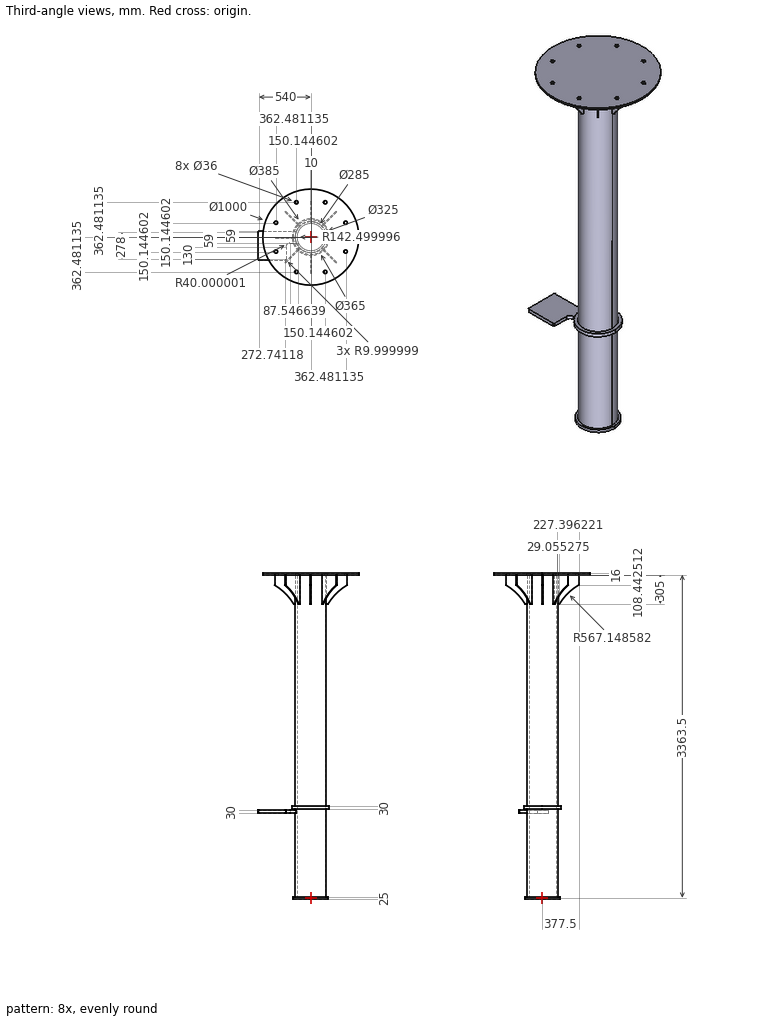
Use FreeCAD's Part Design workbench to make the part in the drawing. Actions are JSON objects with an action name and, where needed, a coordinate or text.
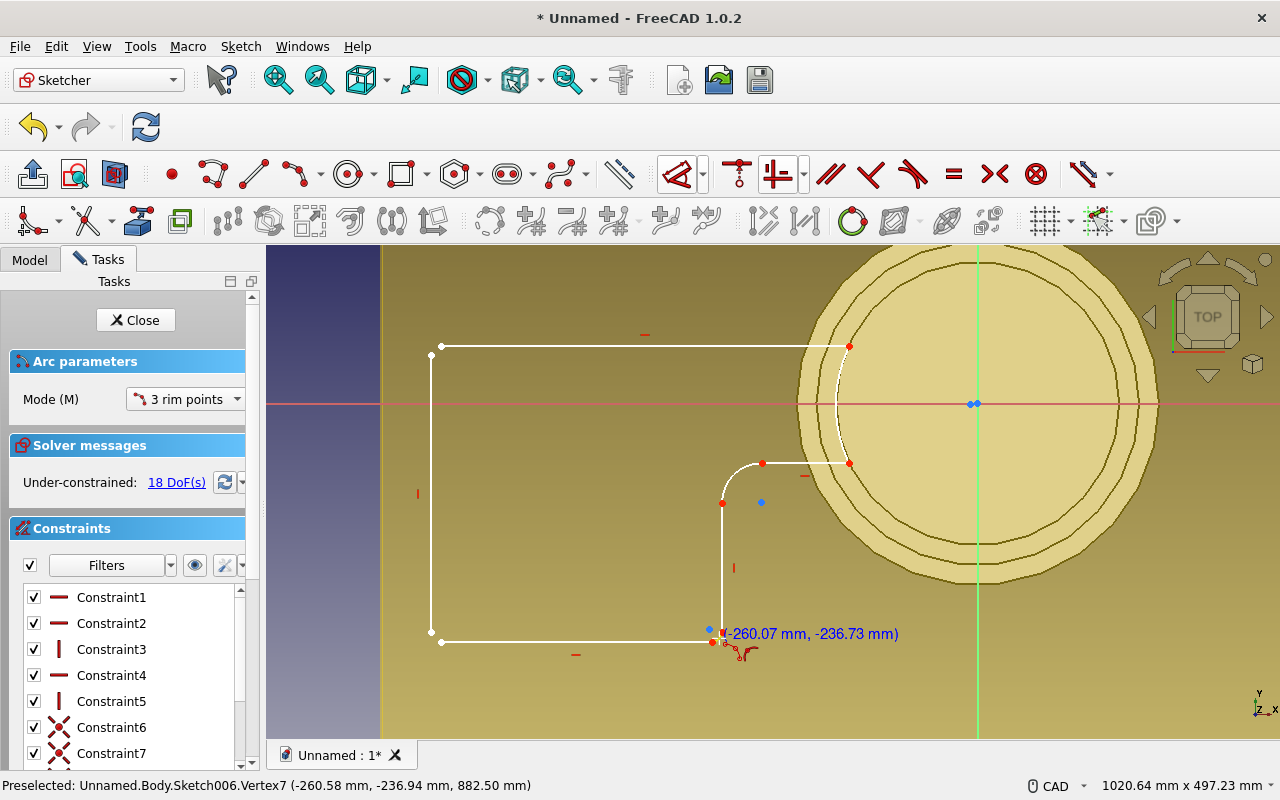
{"action": "left_click", "coordinate": [441, 642]}
{"action": "left_click", "coordinate": [431, 632]}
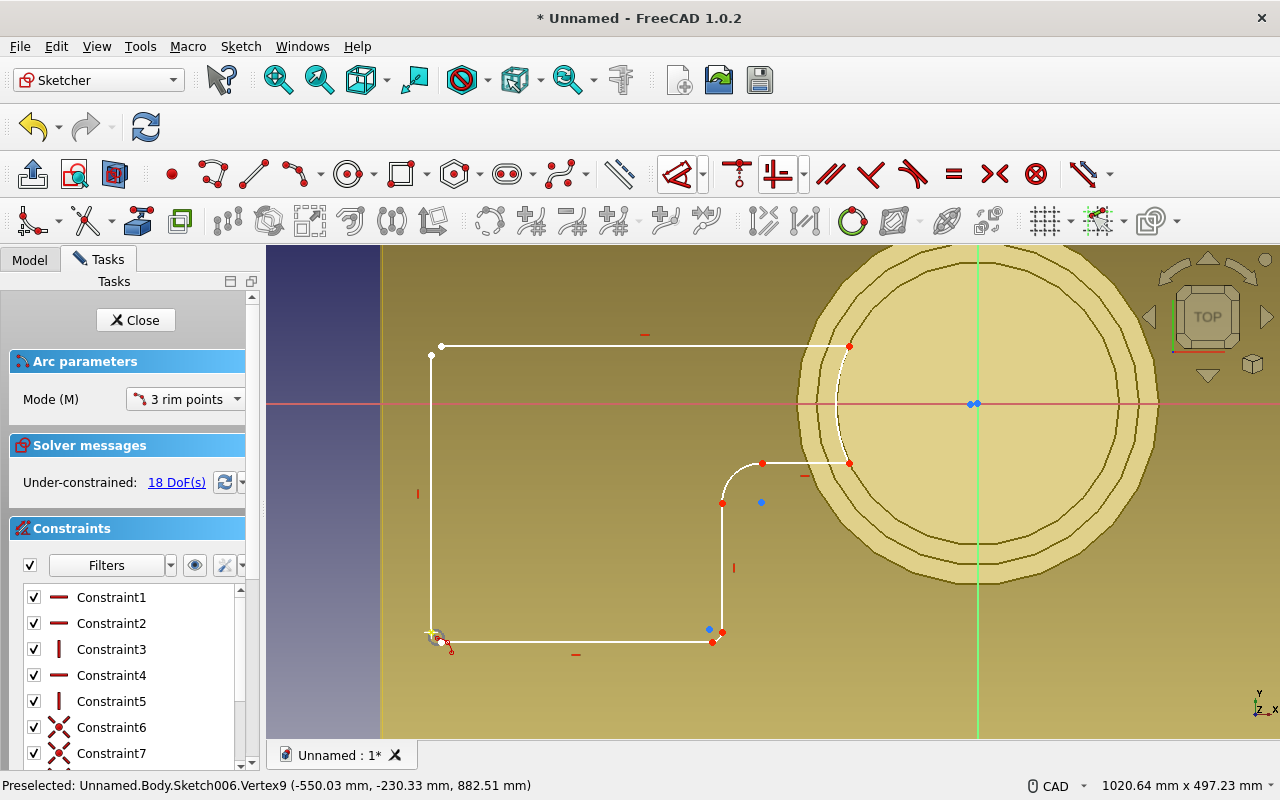
{"action": "scroll", "coordinate": [434, 638], "scroll_direction": "up", "scroll_amount": 9}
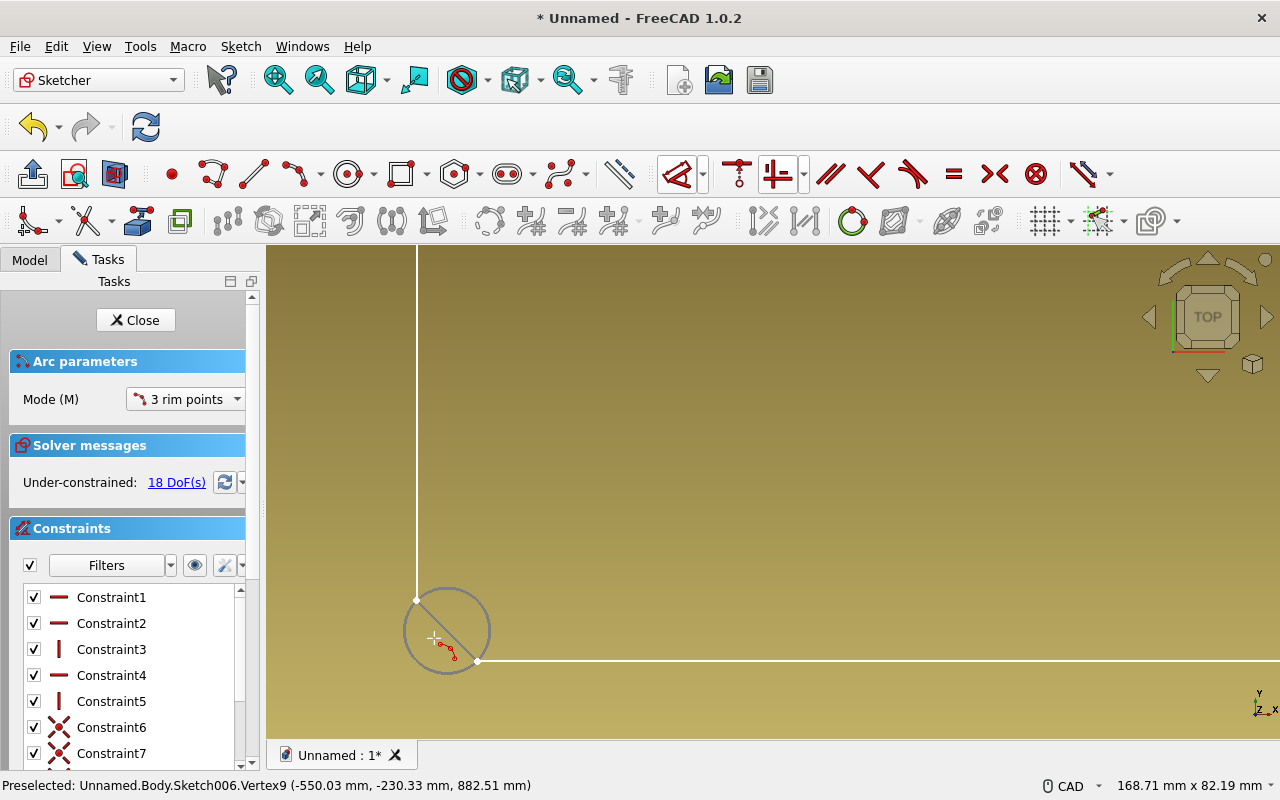
{"action": "left_click", "coordinate": [435, 635]}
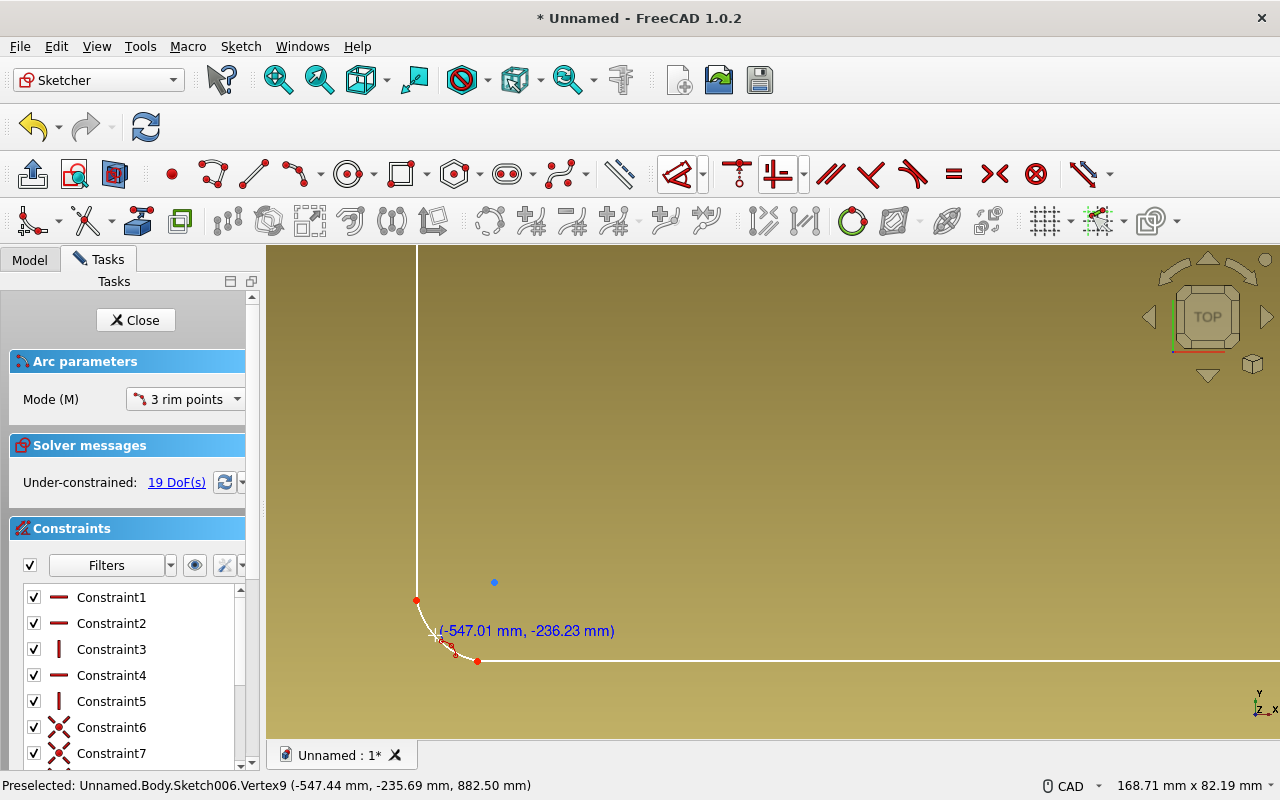
{"action": "scroll", "coordinate": [434, 638], "scroll_direction": "down", "scroll_amount": 9}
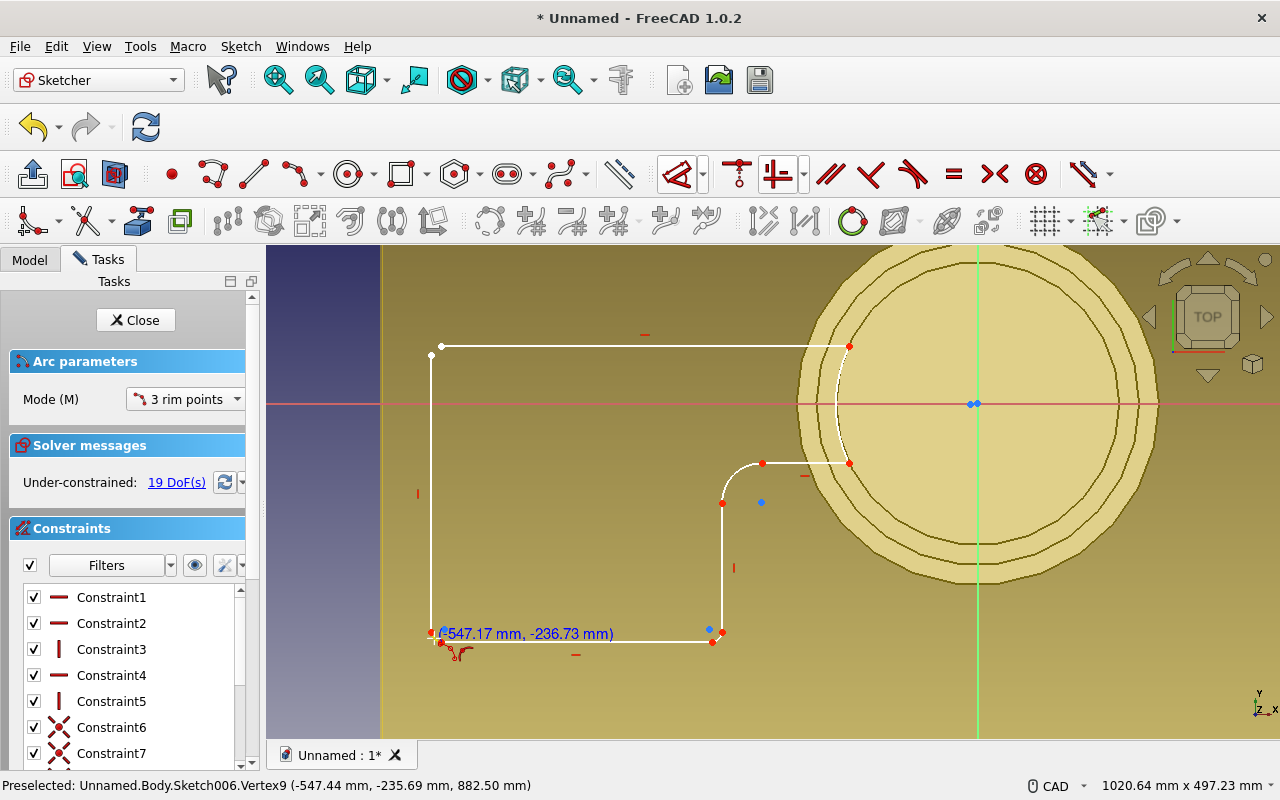
{"action": "left_click", "coordinate": [431, 355]}
{"action": "left_click", "coordinate": [441, 346]}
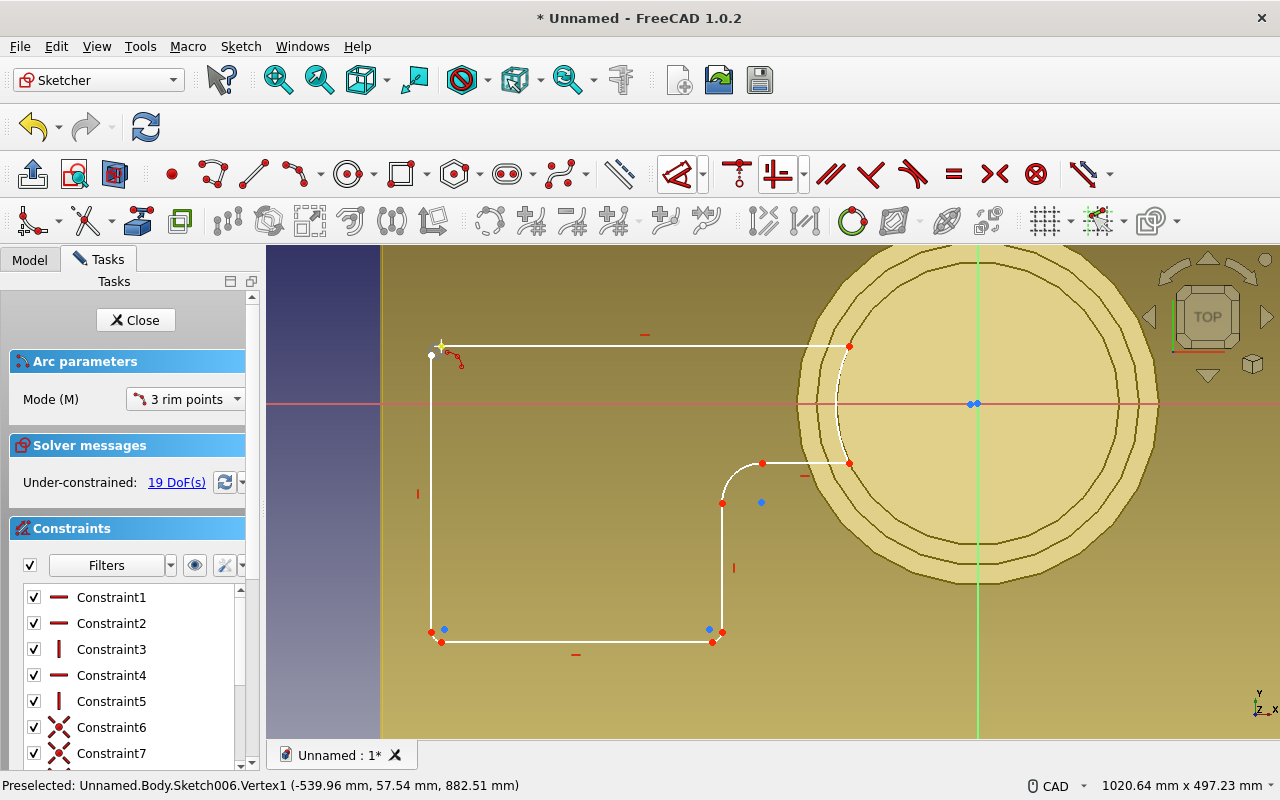
{"action": "scroll", "coordinate": [434, 348], "scroll_direction": "up", "scroll_amount": 9}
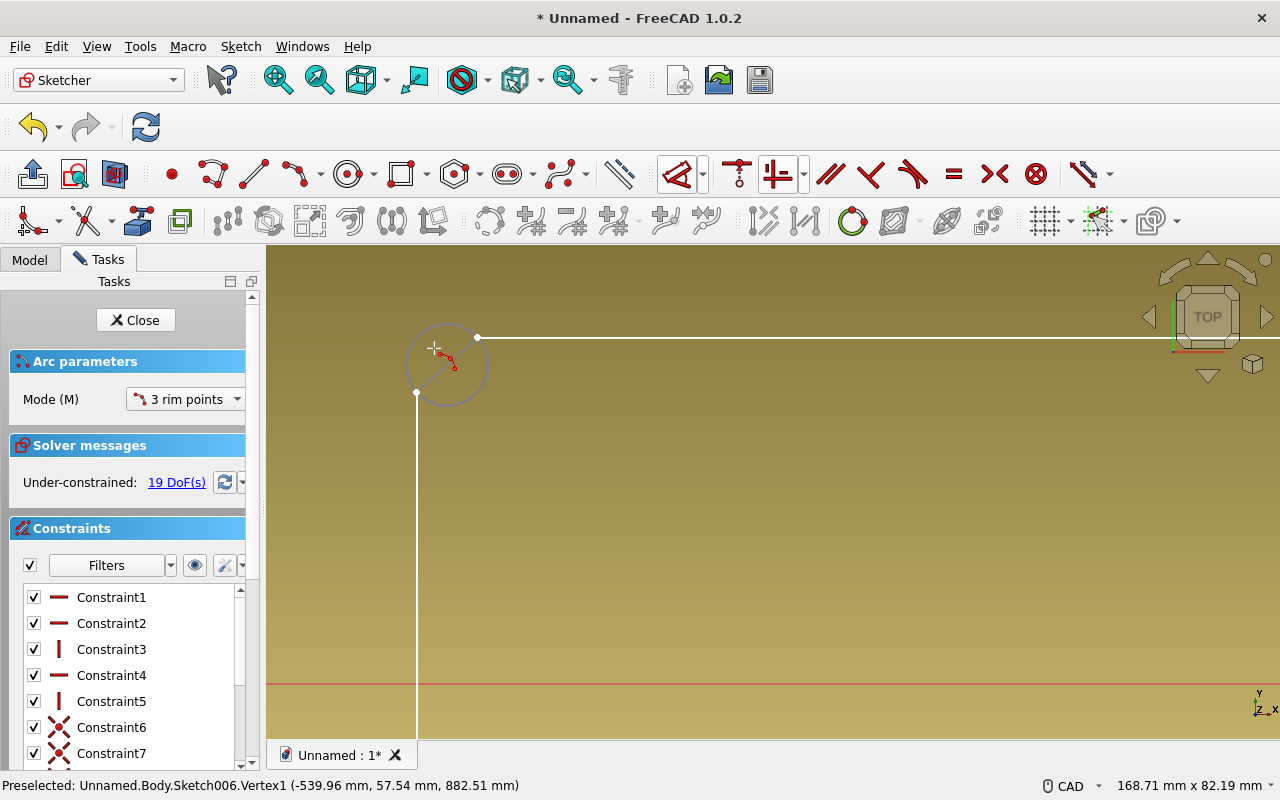
{"action": "left_click", "coordinate": [435, 347]}
{"action": "key", "text": "Escape"}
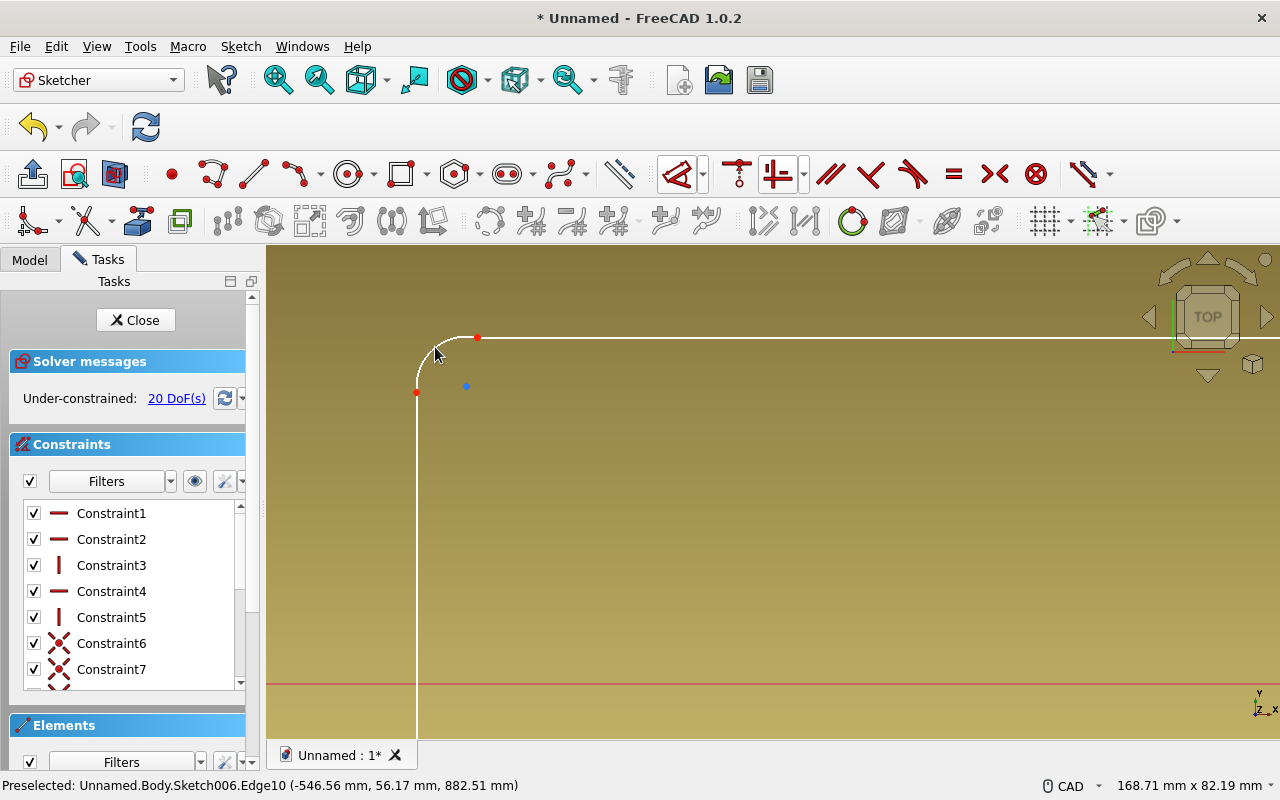
{"action": "scroll", "coordinate": [434, 347], "scroll_direction": "down", "scroll_amount": 9}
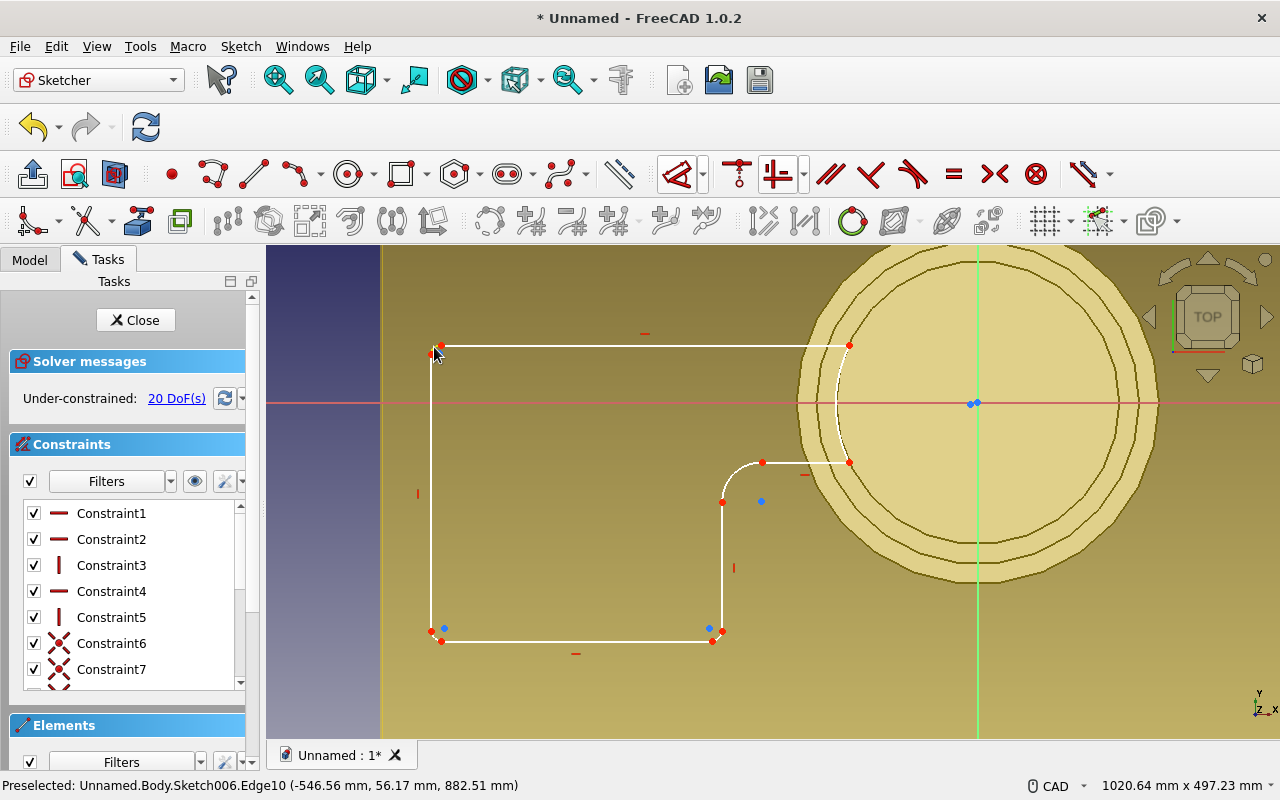
{"action": "left_click", "coordinate": [523, 346]}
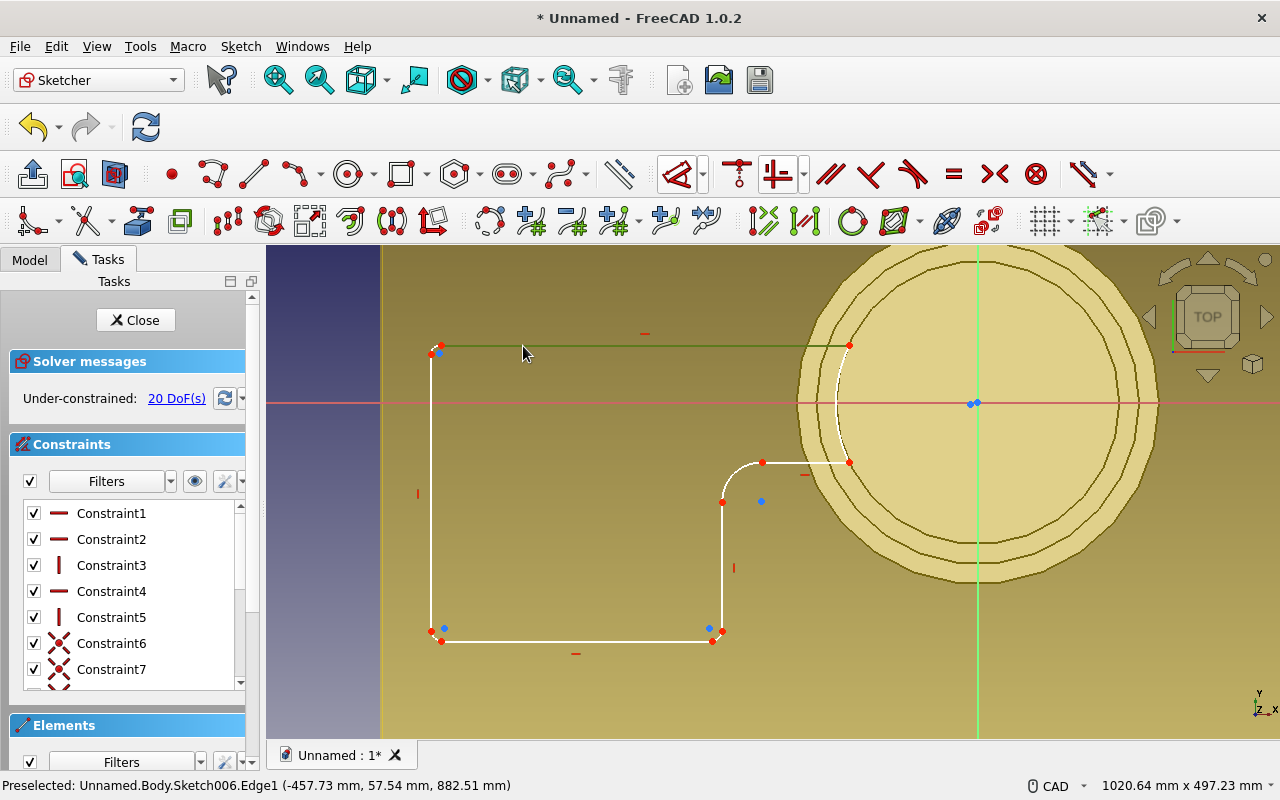
{"action": "scroll", "coordinate": [434, 348], "scroll_direction": "up", "scroll_amount": 4}